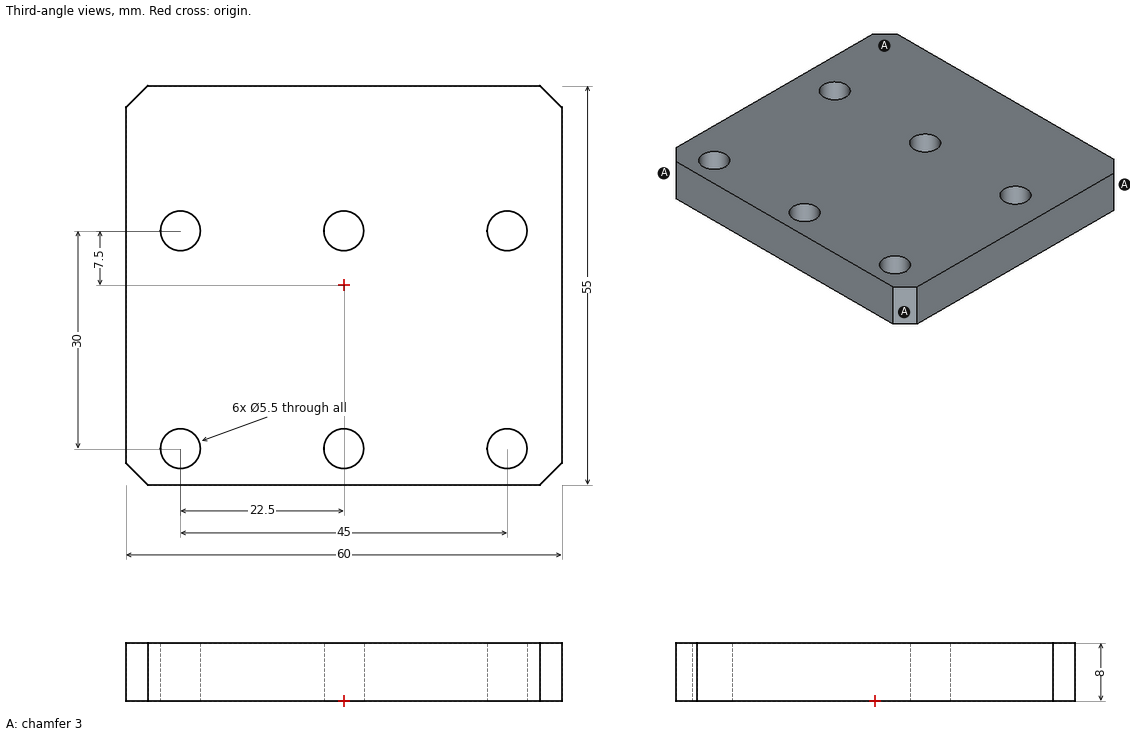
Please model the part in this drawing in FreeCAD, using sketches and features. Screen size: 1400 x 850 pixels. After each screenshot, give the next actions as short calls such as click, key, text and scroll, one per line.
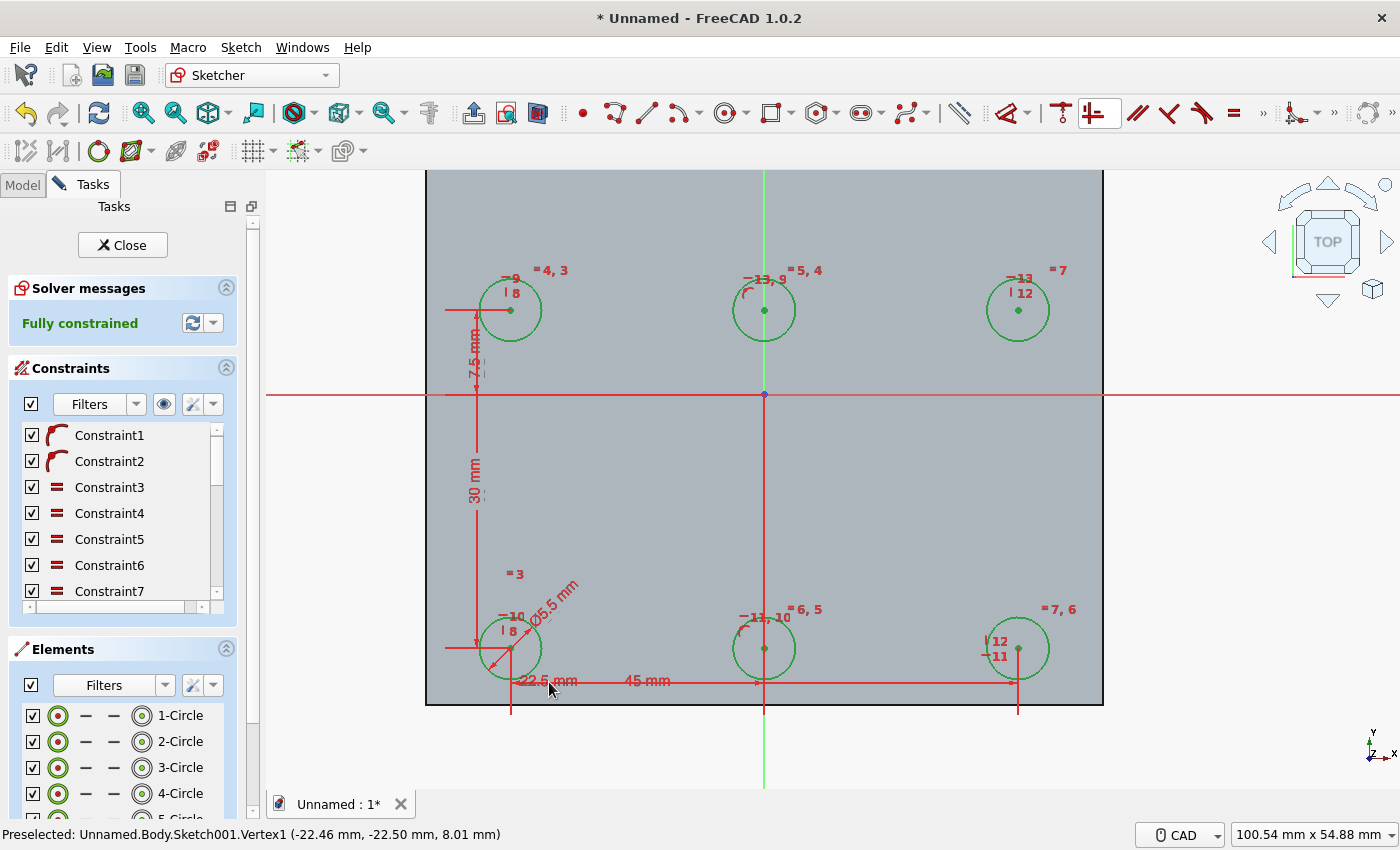
click(123, 245)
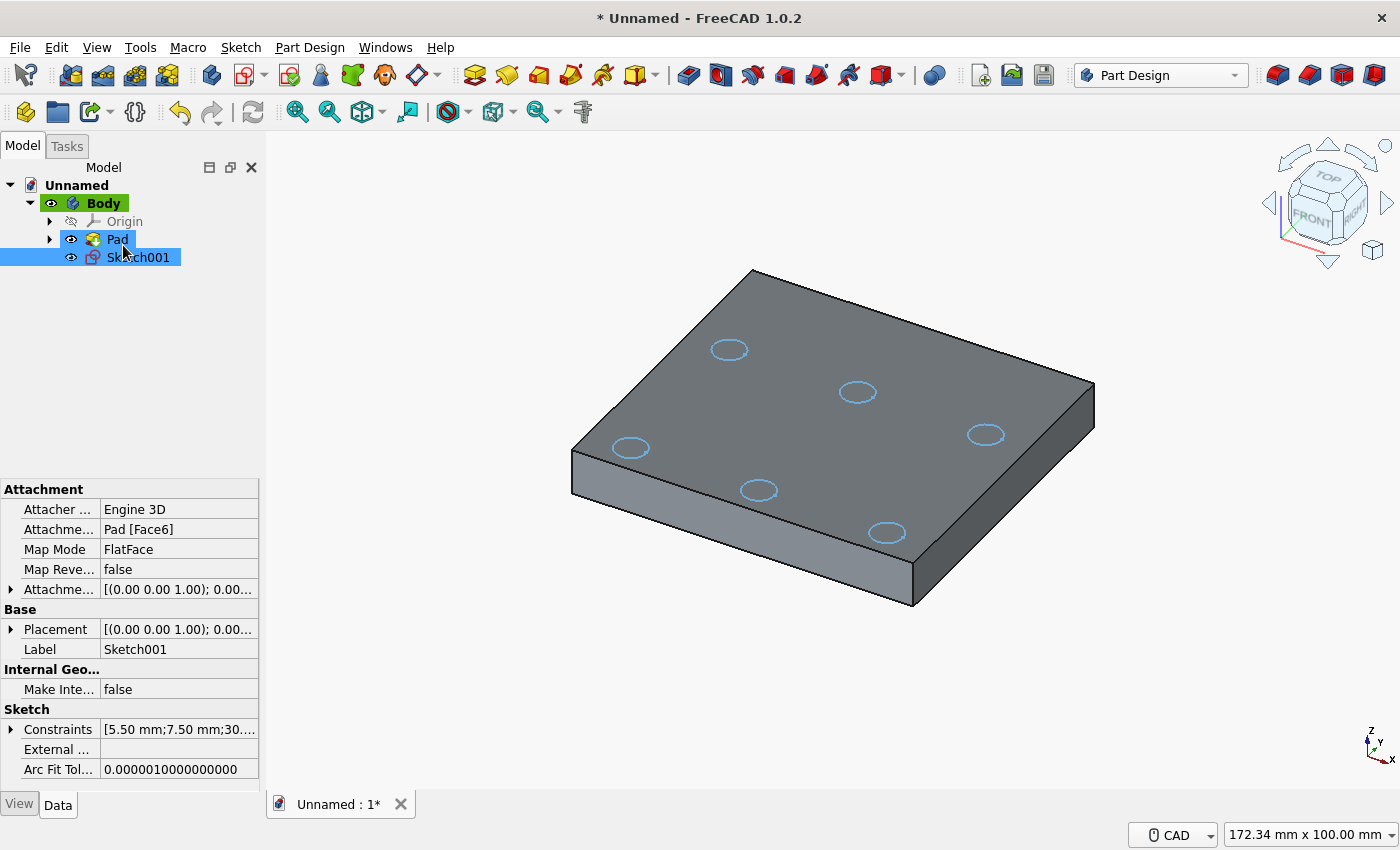
click(722, 76)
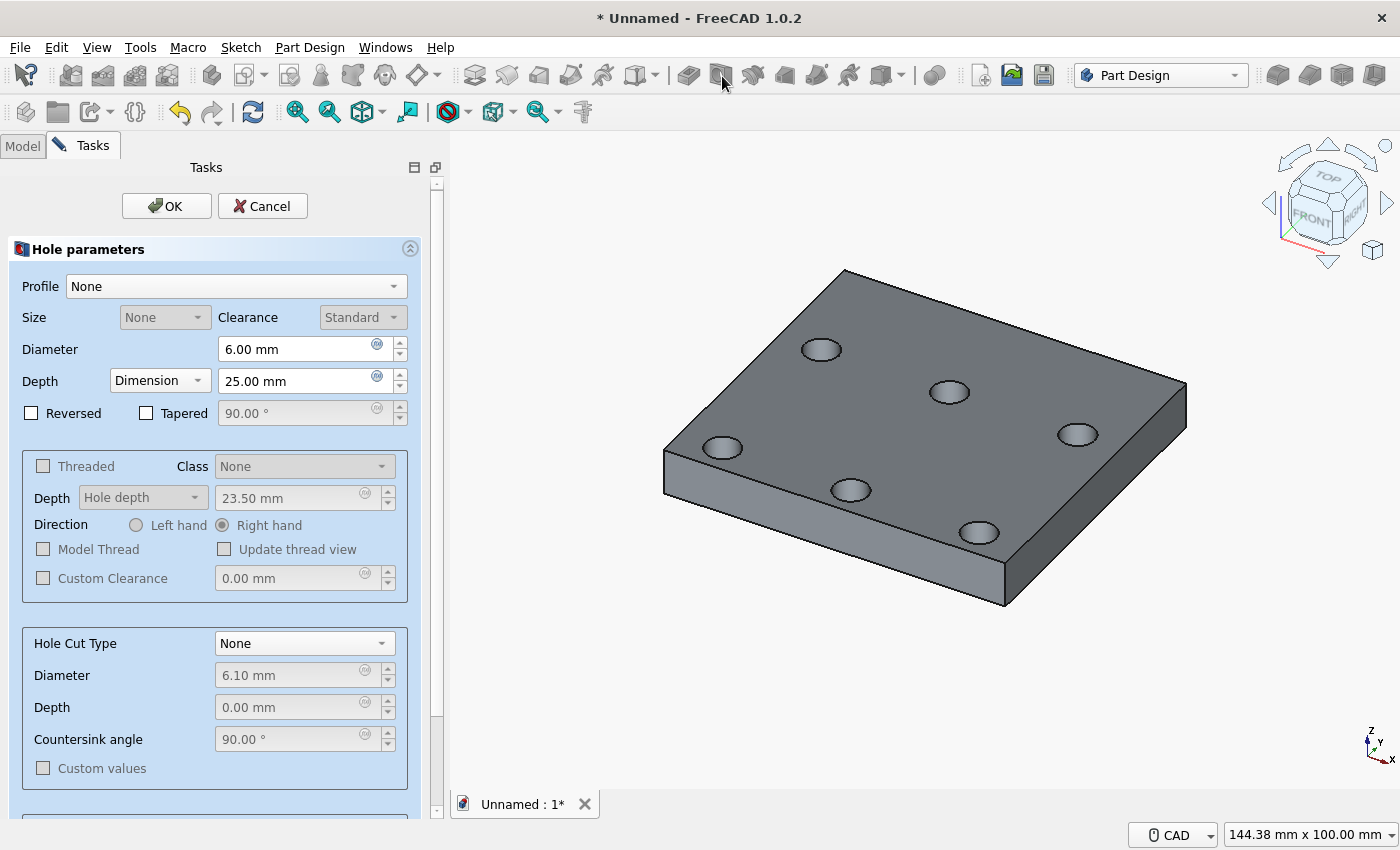
triple_click(305, 349)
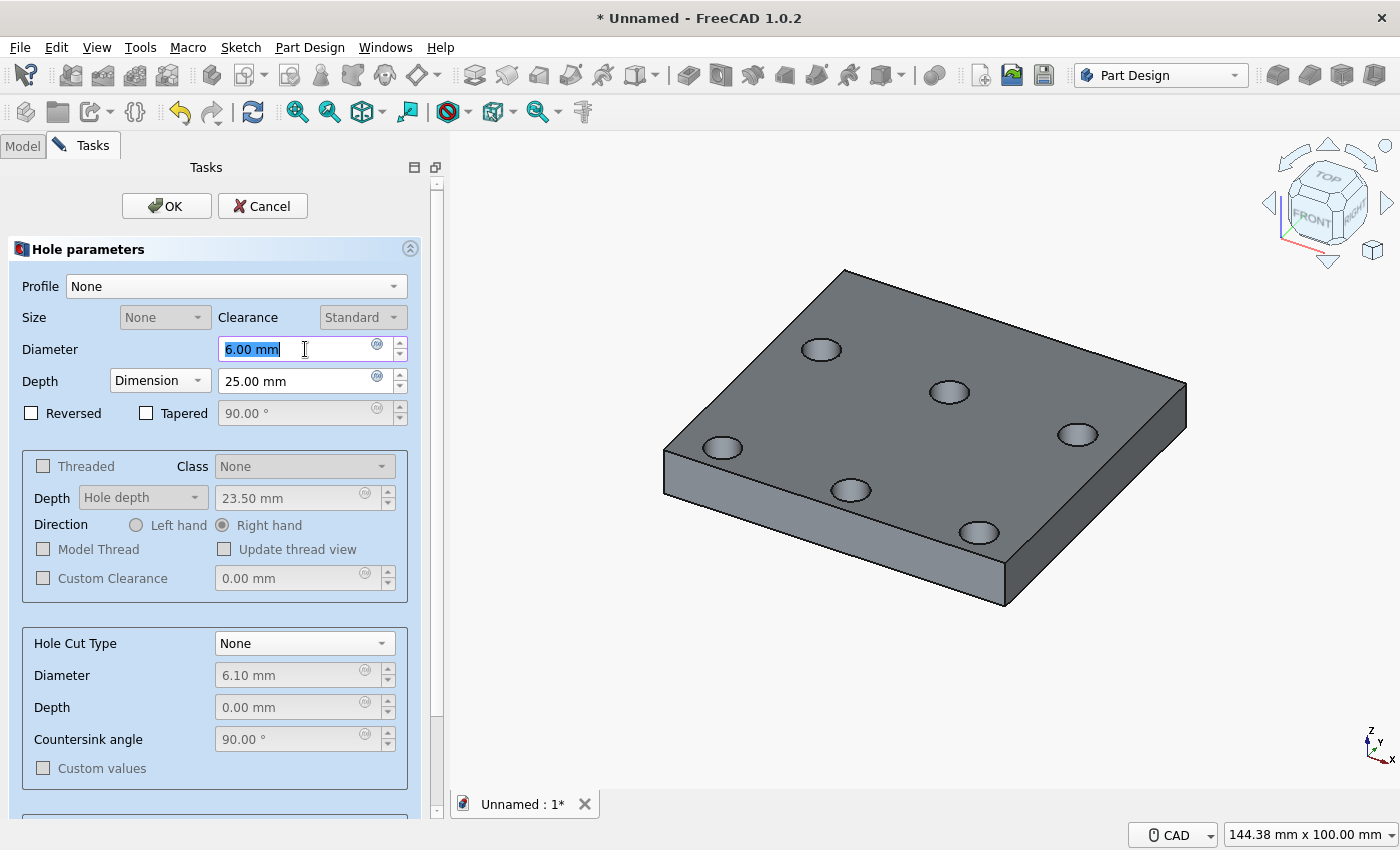
text(5.5)
key(Tab)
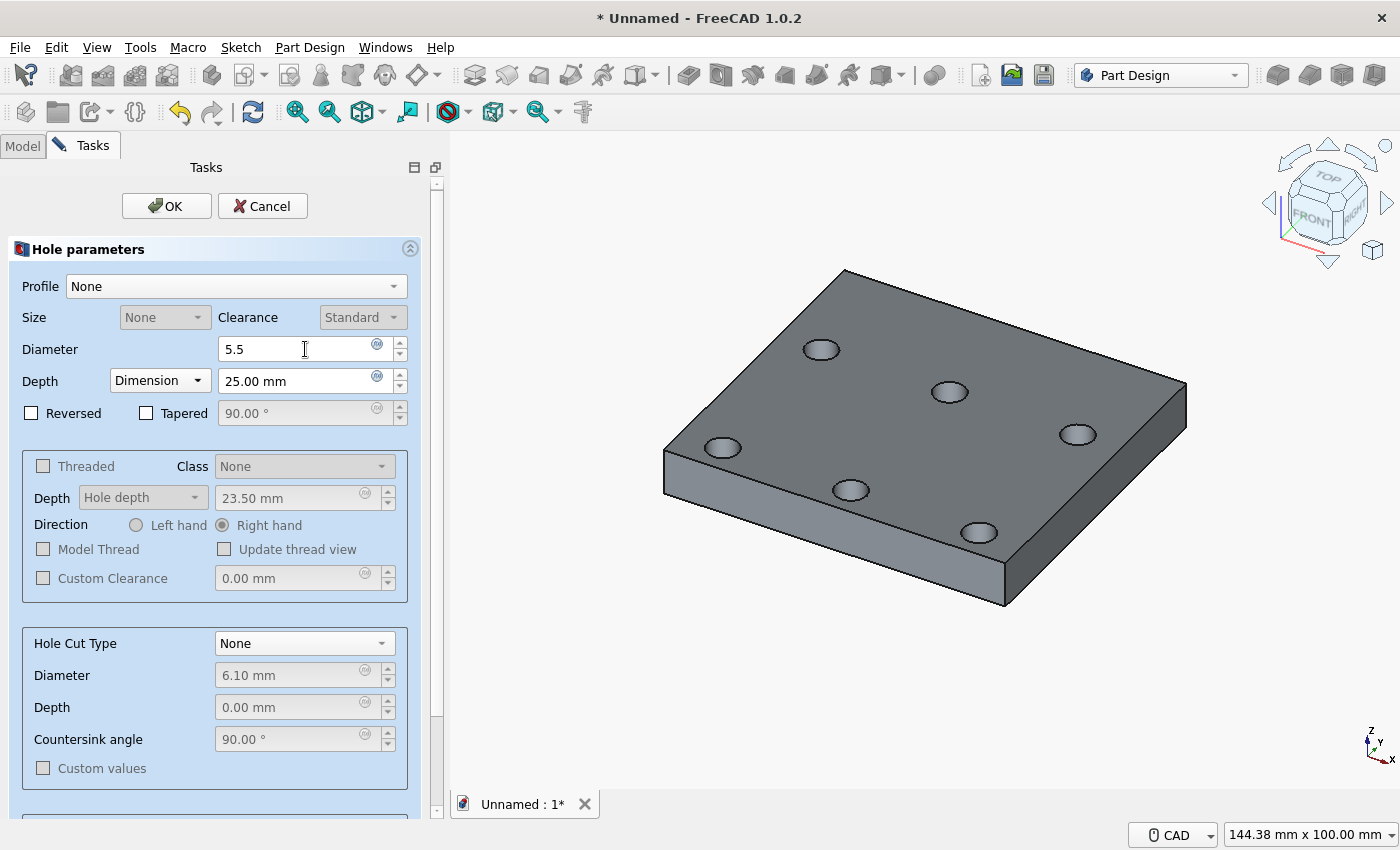
click(161, 380)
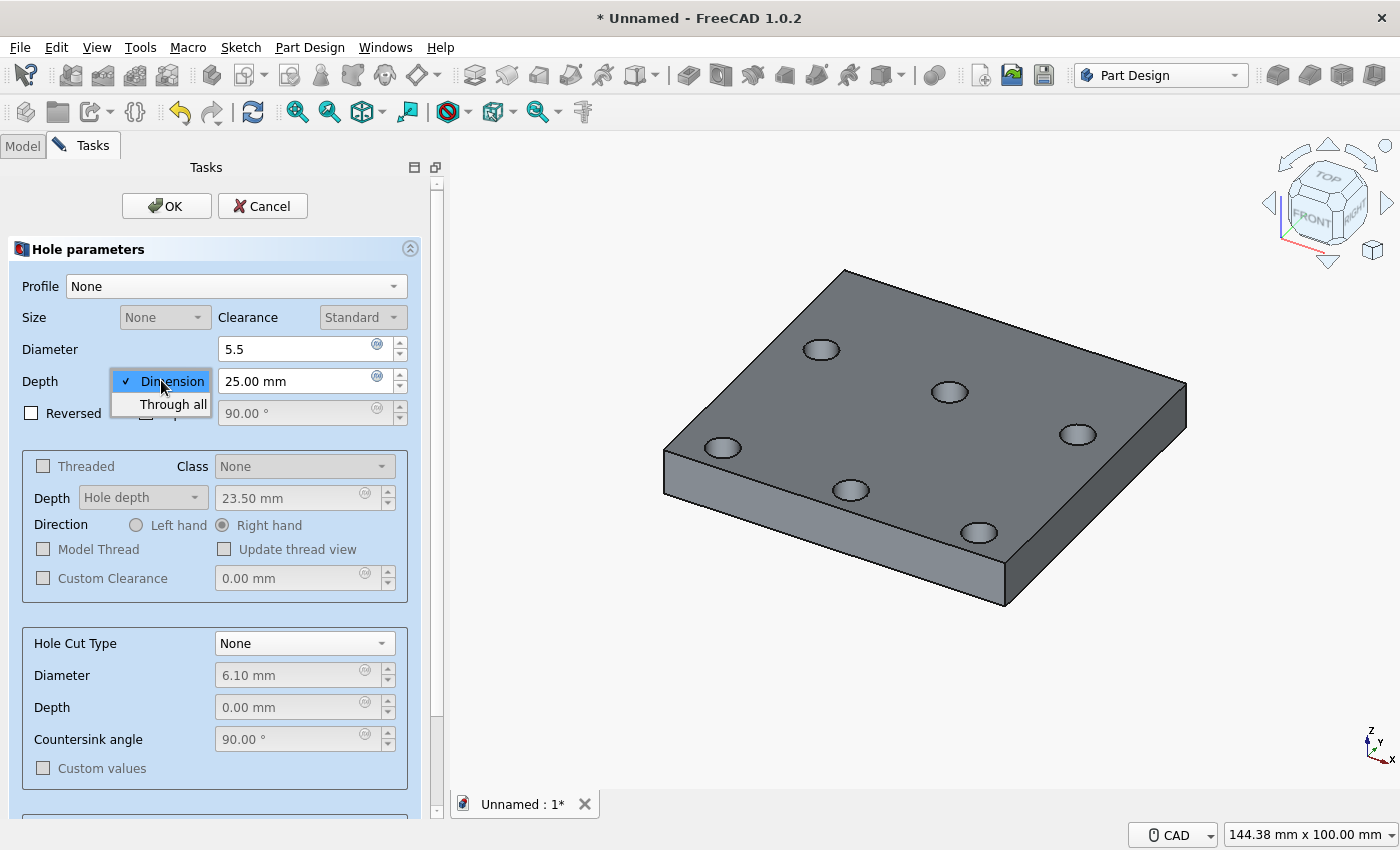
click(160, 404)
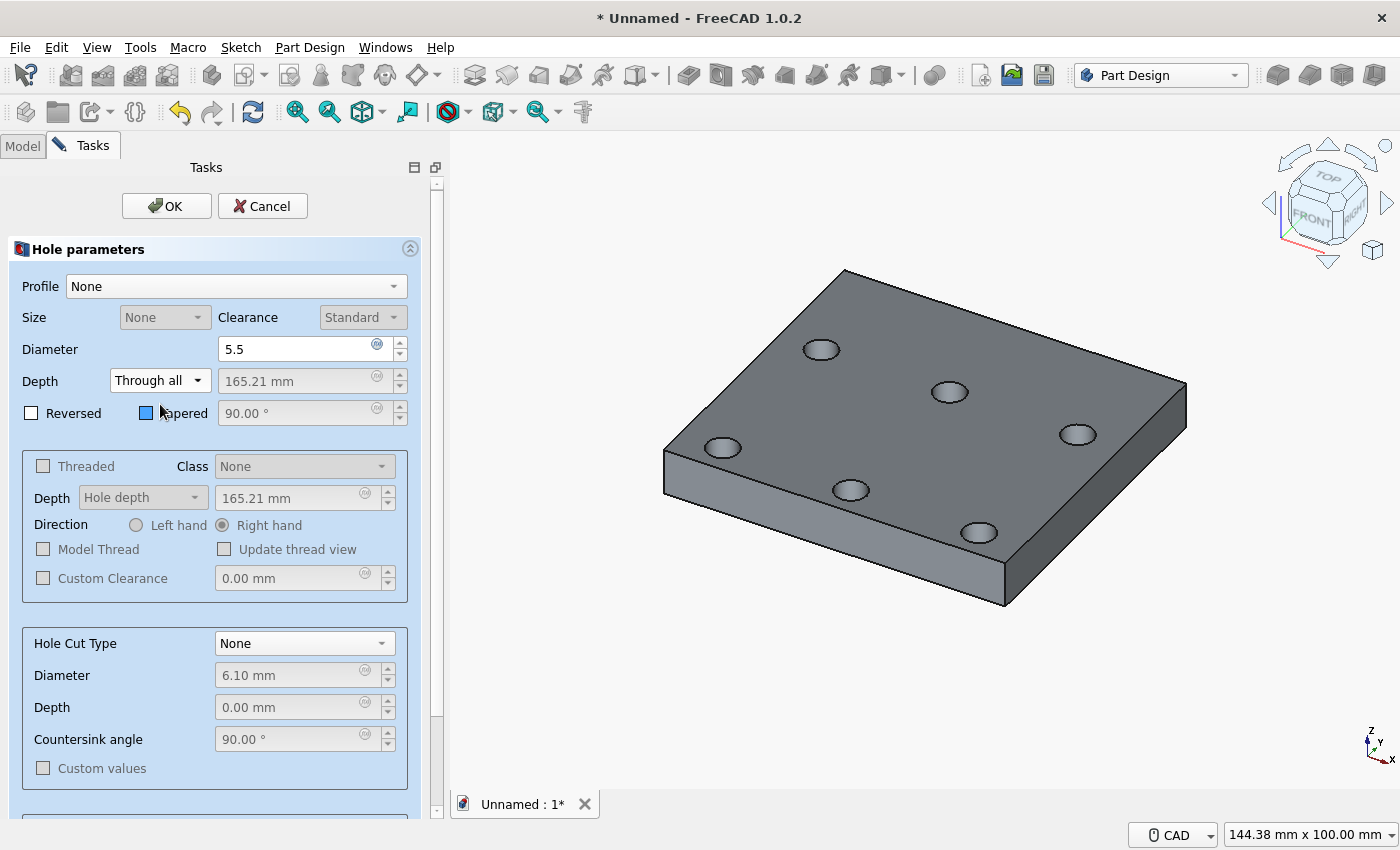
click(167, 206)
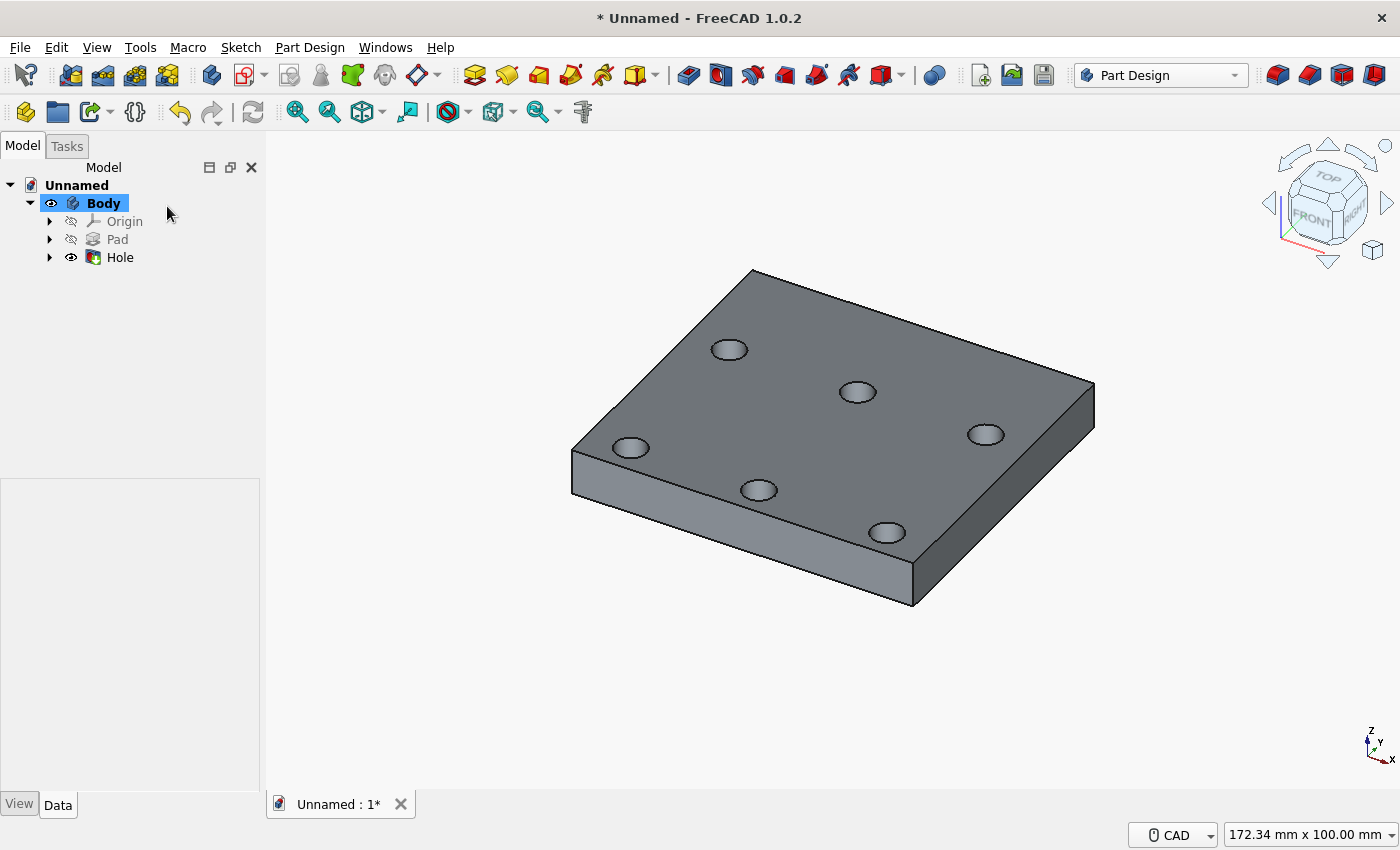
click(913, 584)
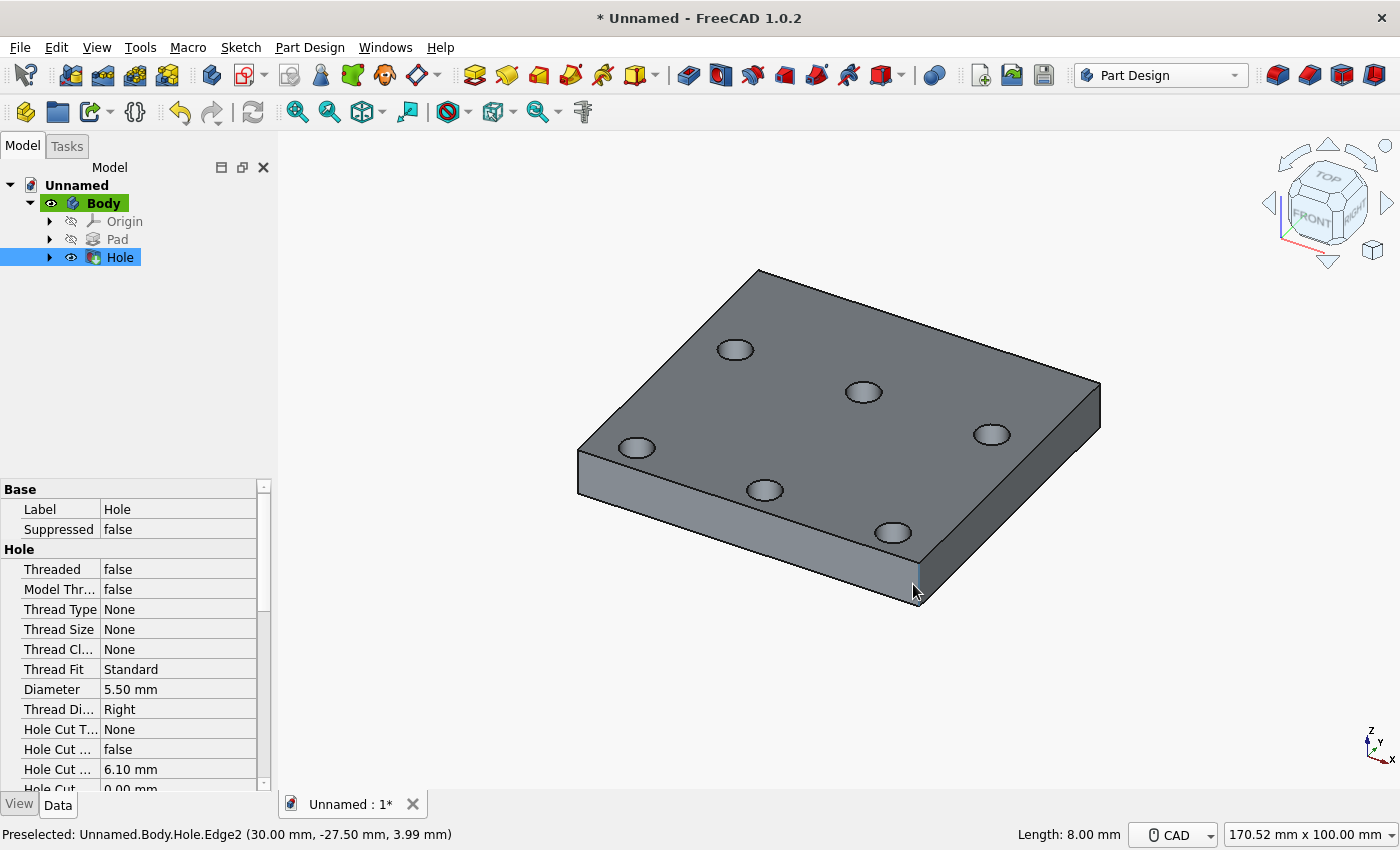
key(0)